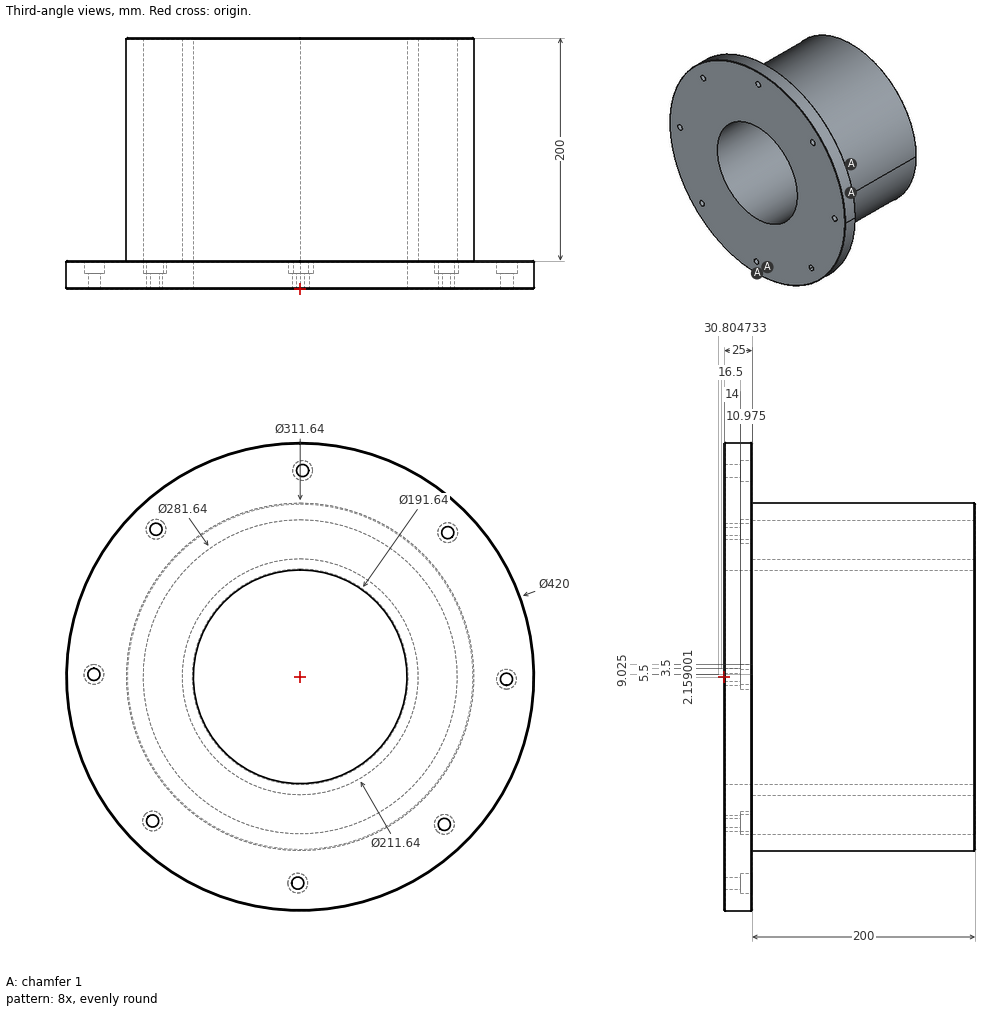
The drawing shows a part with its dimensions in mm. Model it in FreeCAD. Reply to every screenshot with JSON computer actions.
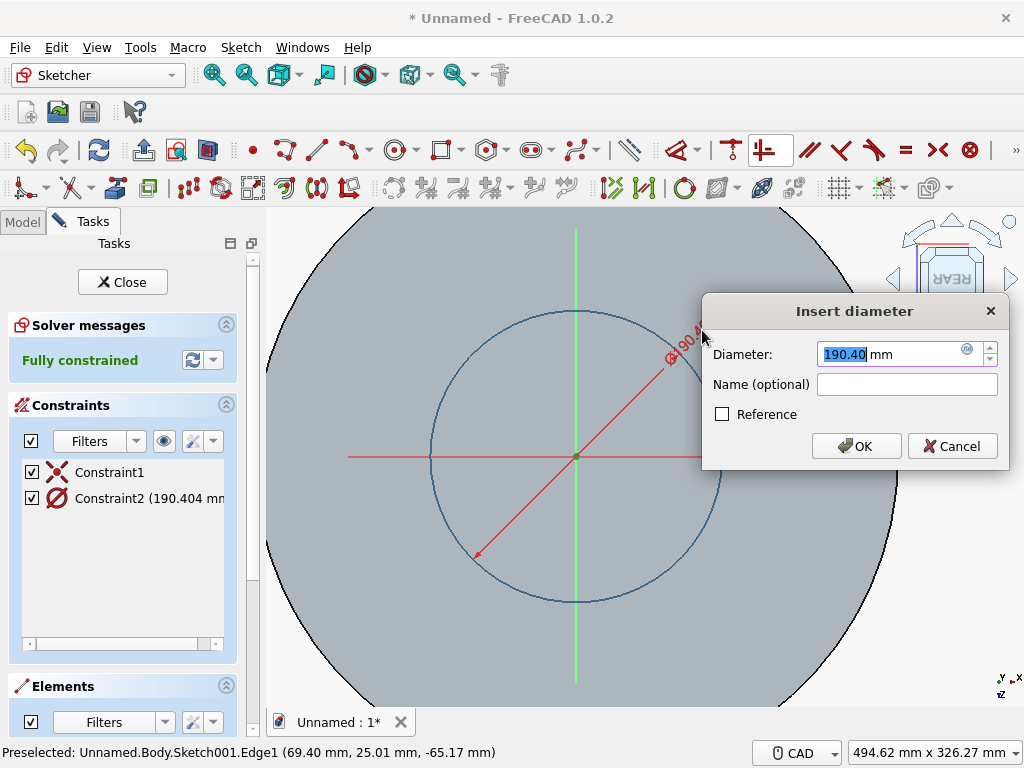
{"action": "type", "text": "191.64"}
{"action": "key", "text": "Return"}
{"action": "key", "text": "Escape"}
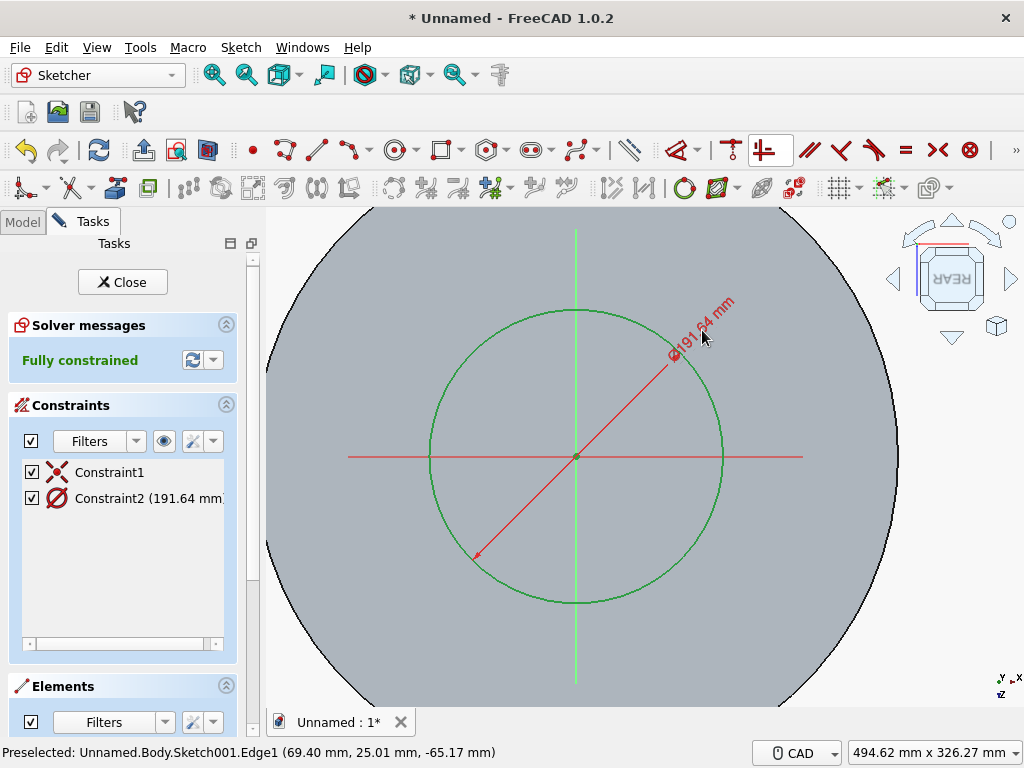
{"action": "left_click", "coordinate": [123, 282]}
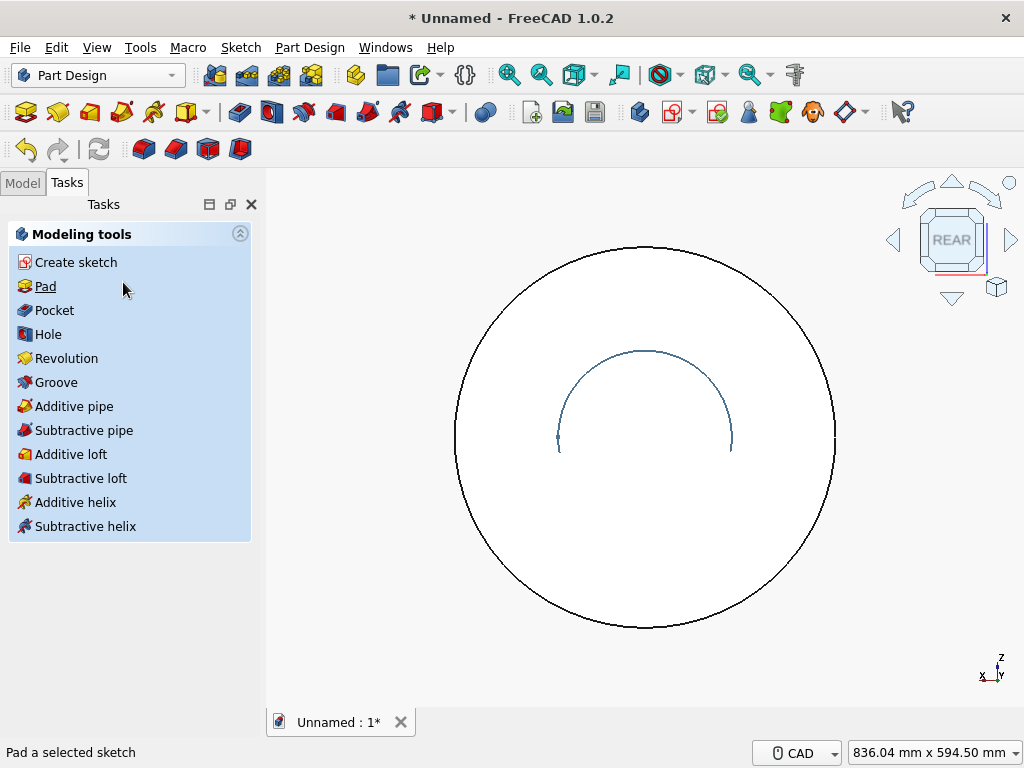
{"action": "left_click", "coordinate": [240, 112]}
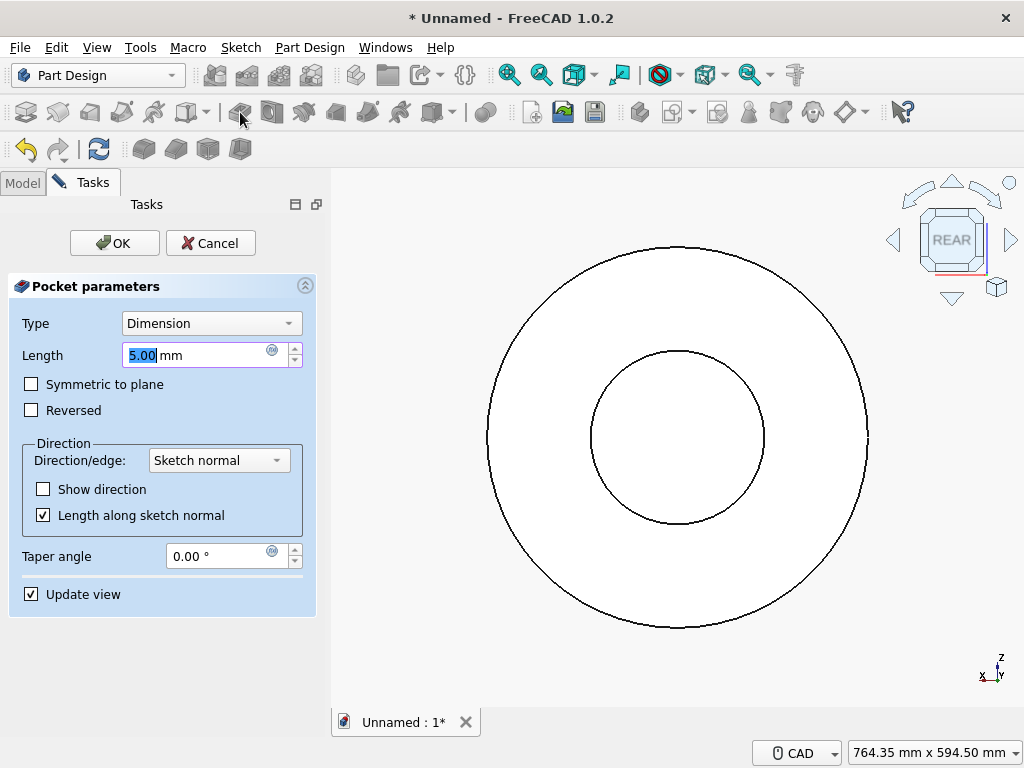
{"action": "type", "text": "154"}
{"action": "key", "text": "Tab"}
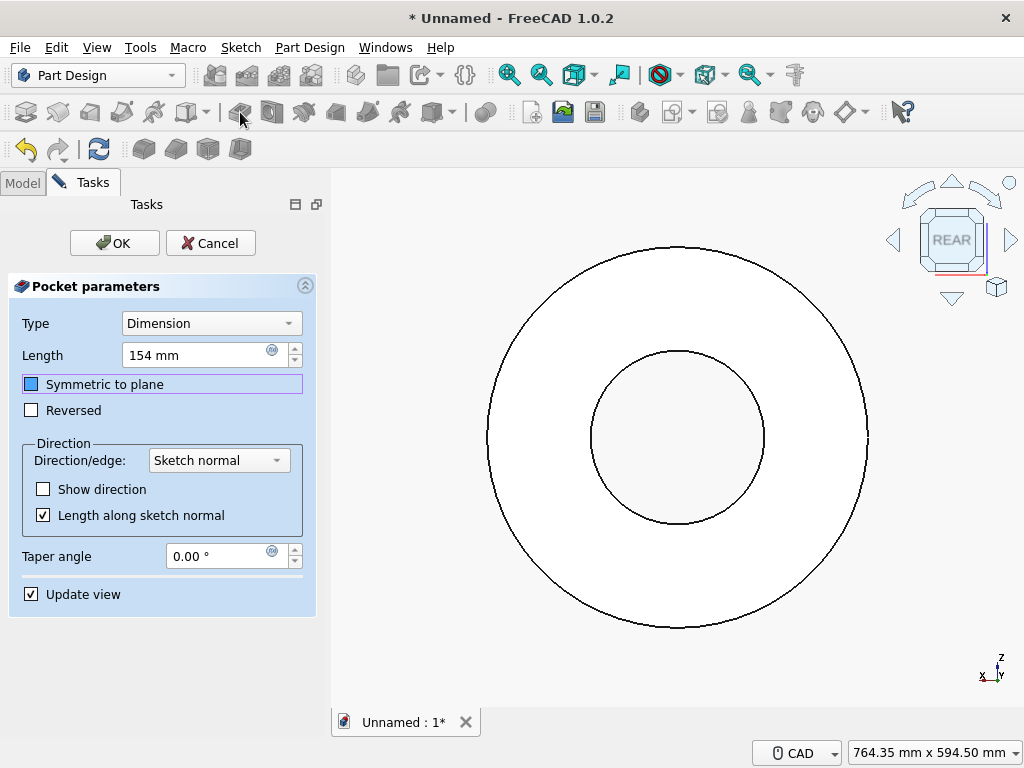
{"action": "left_click", "coordinate": [115, 243]}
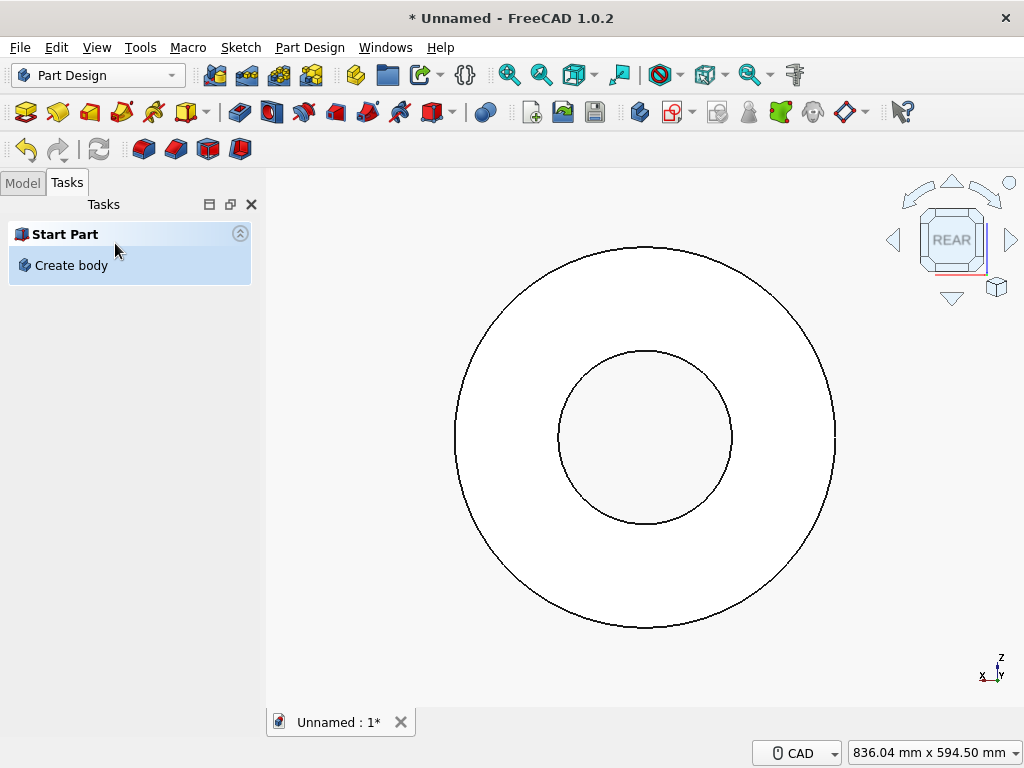
{"action": "left_click", "coordinate": [23, 182]}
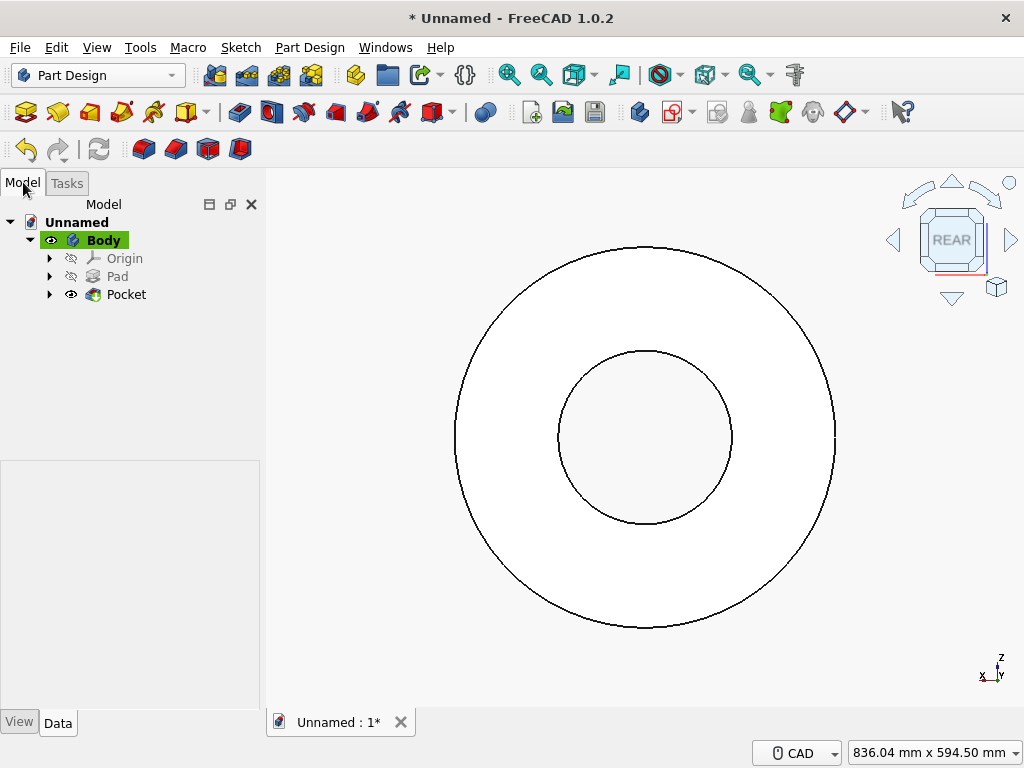
{"action": "left_click", "coordinate": [50, 258]}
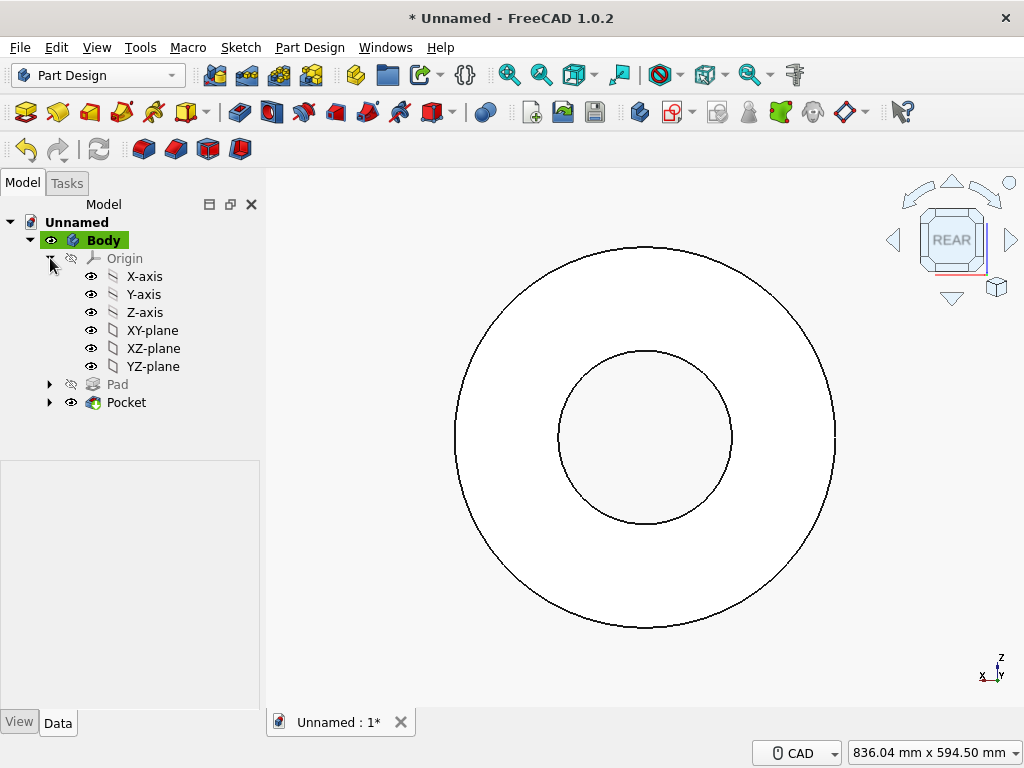
{"action": "left_click", "coordinate": [136, 348]}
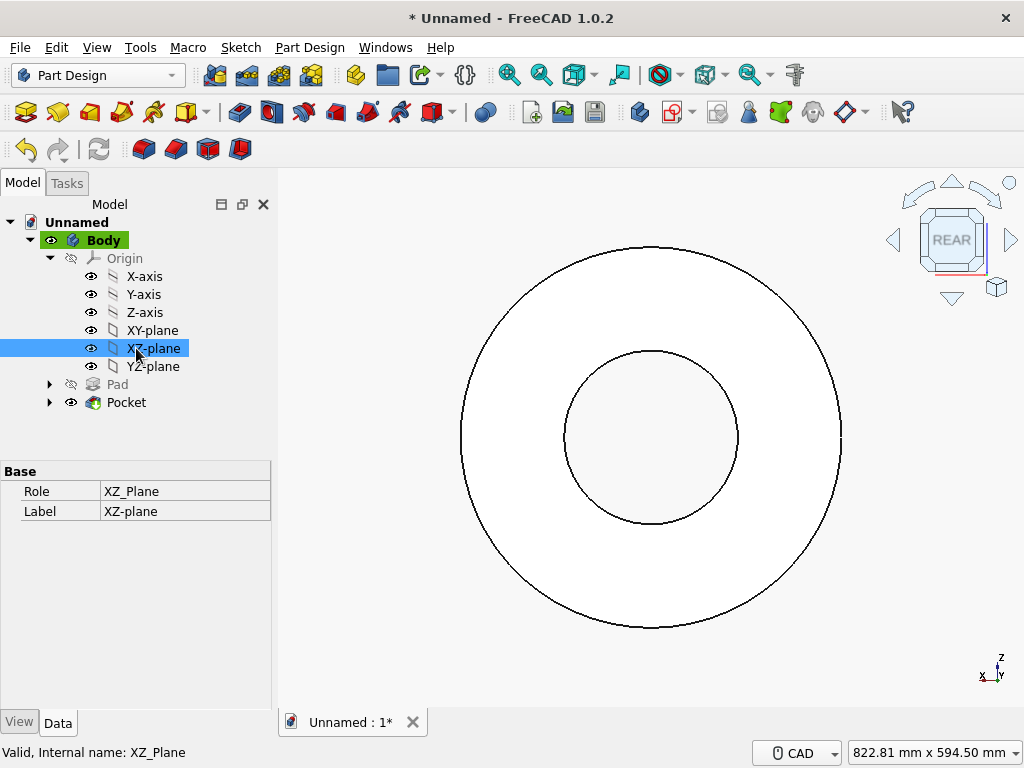
{"action": "left_click", "coordinate": [846, 112]}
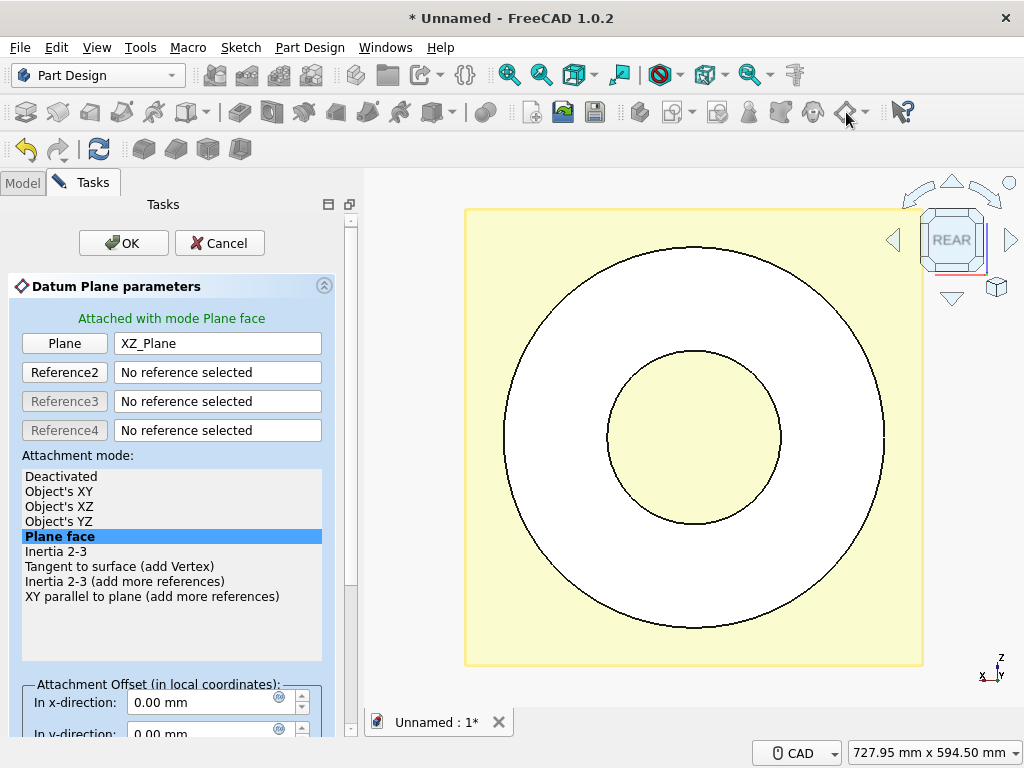
{"action": "scroll", "coordinate": [351, 475], "scroll_direction": "down", "scroll_amount": 2}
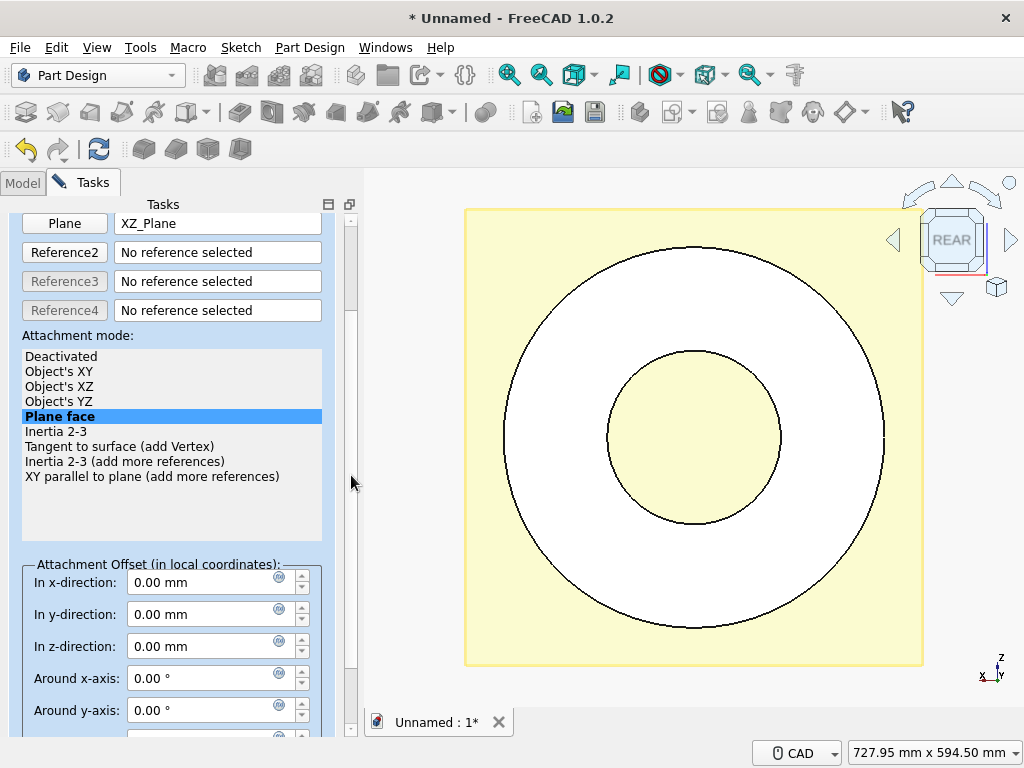
{"action": "triple_click", "coordinate": [210, 646]}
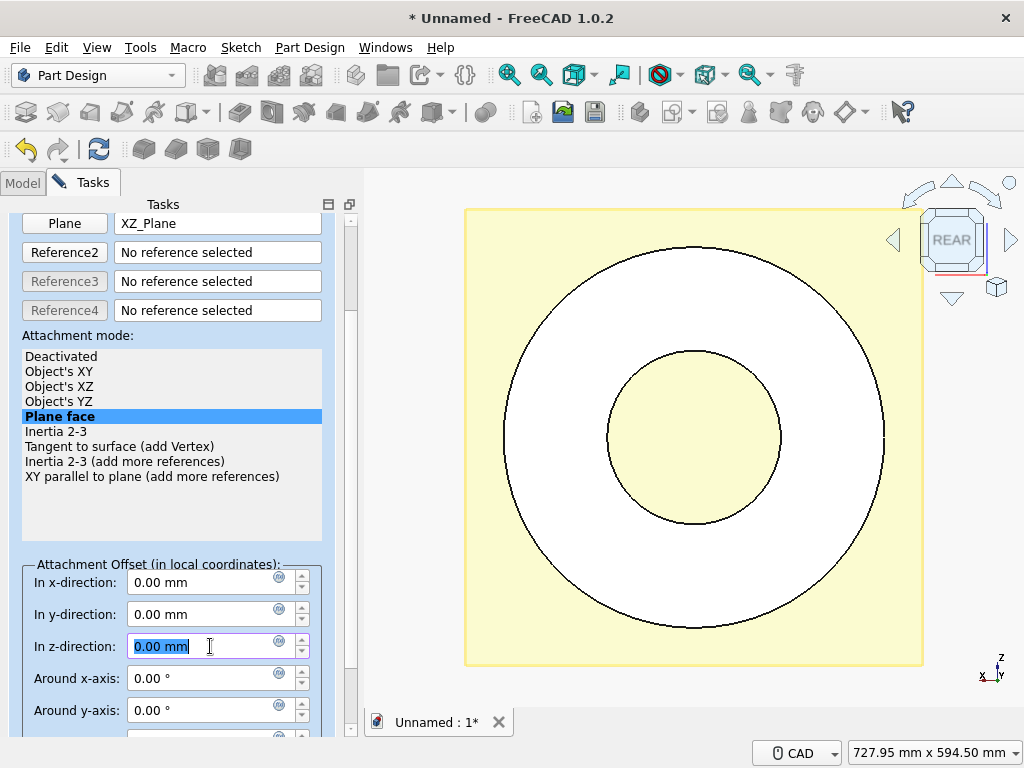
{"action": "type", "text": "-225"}
{"action": "key", "text": "Tab"}